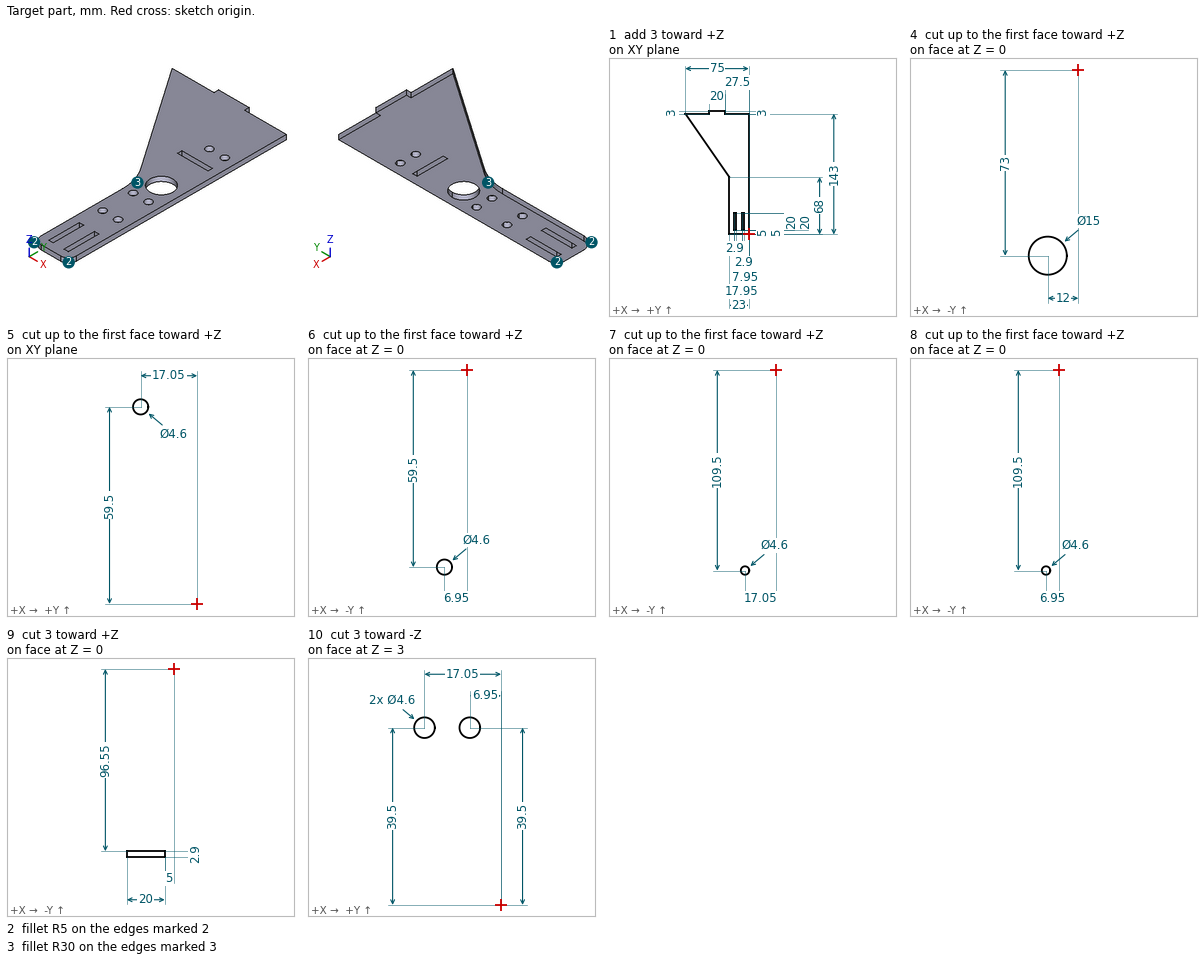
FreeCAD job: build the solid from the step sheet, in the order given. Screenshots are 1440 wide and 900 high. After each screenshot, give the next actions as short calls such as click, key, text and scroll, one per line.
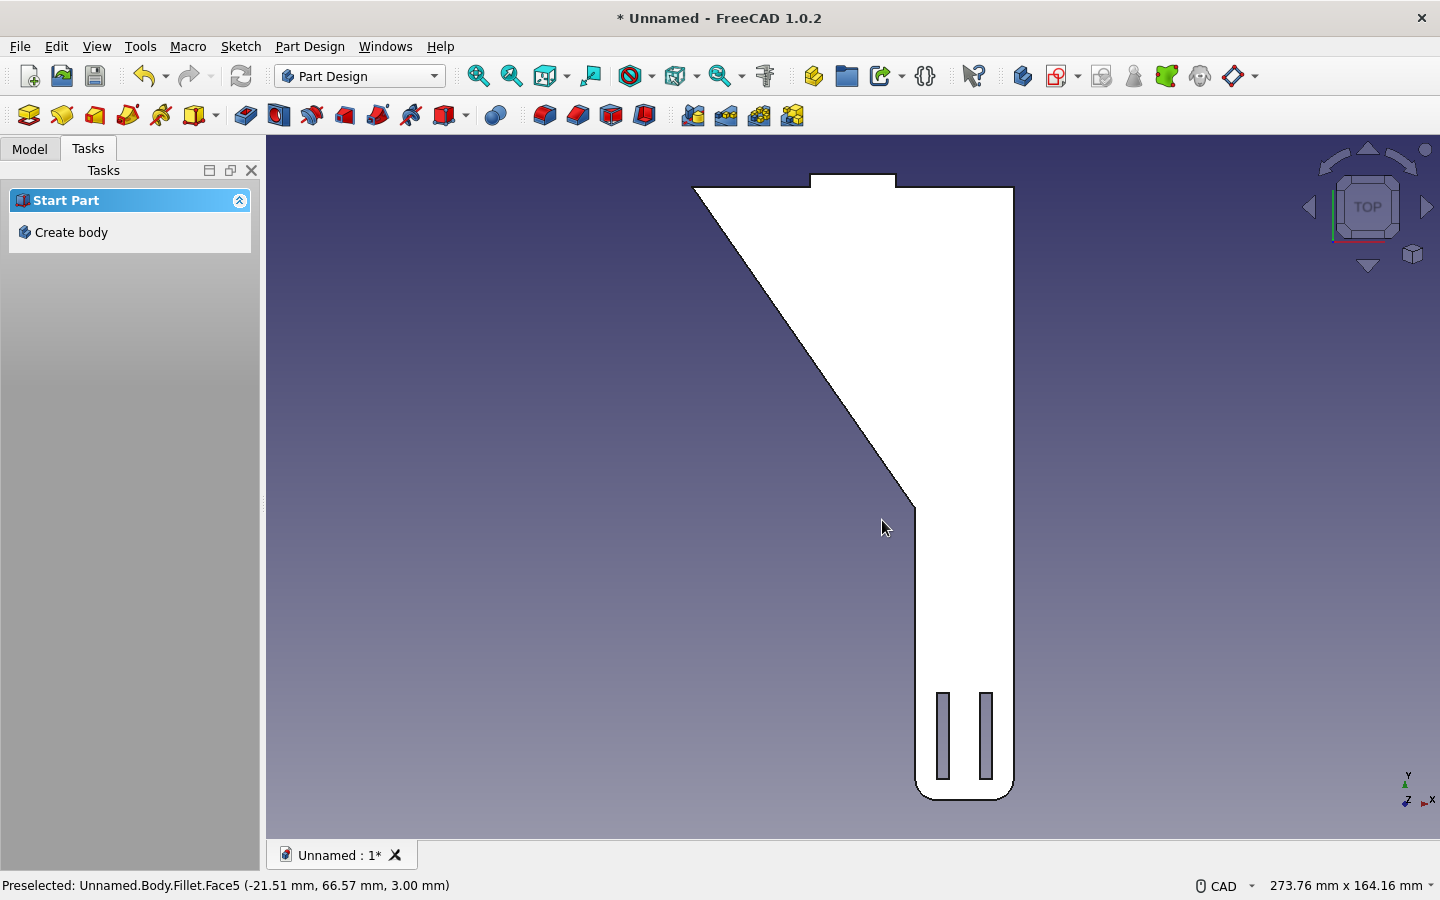
scroll(915, 507, up, 6)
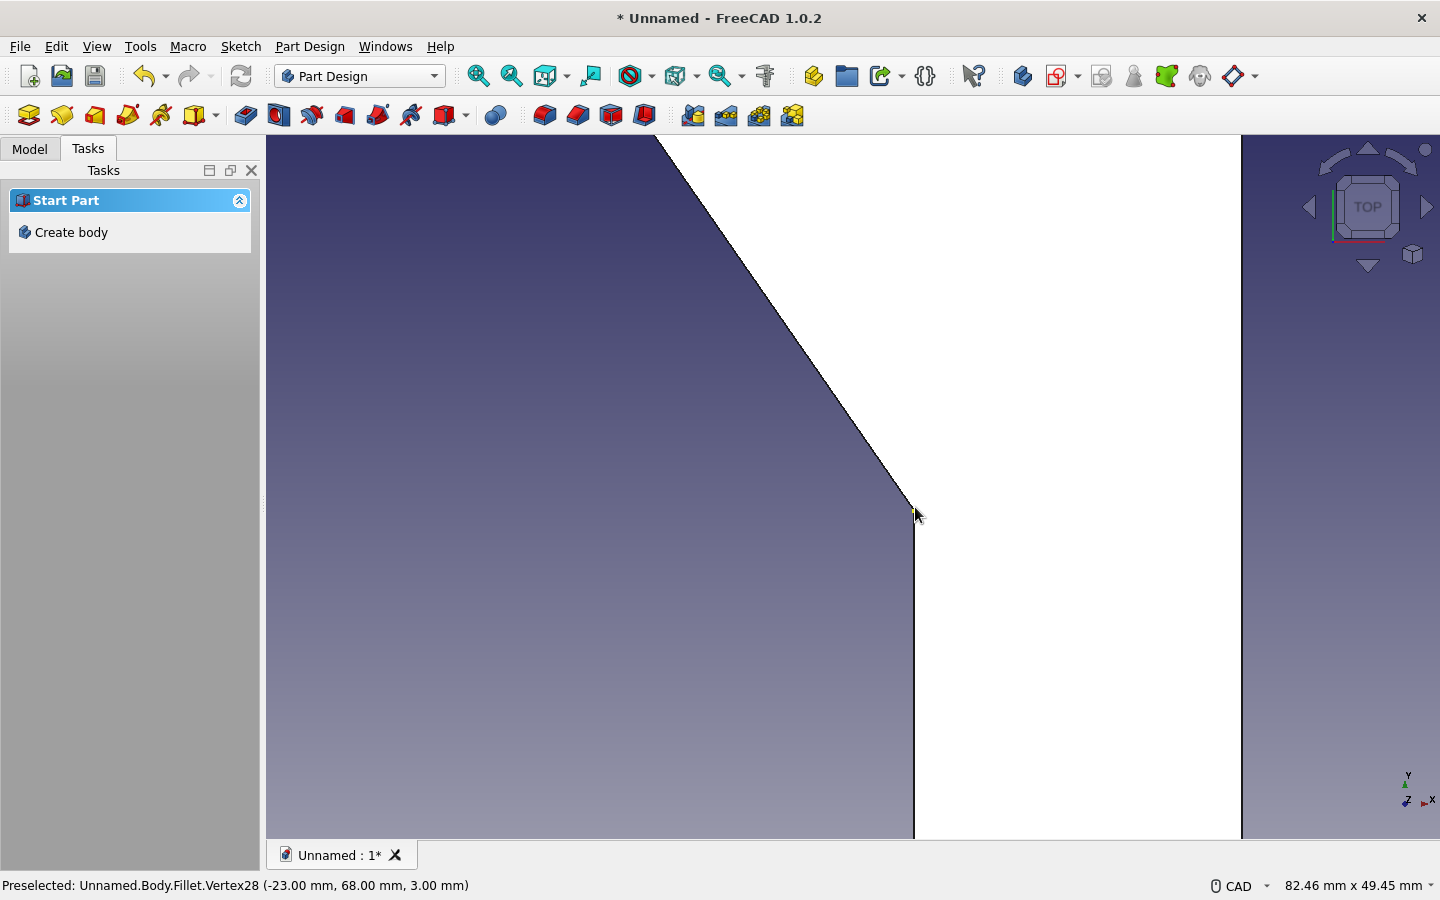
click(479, 76)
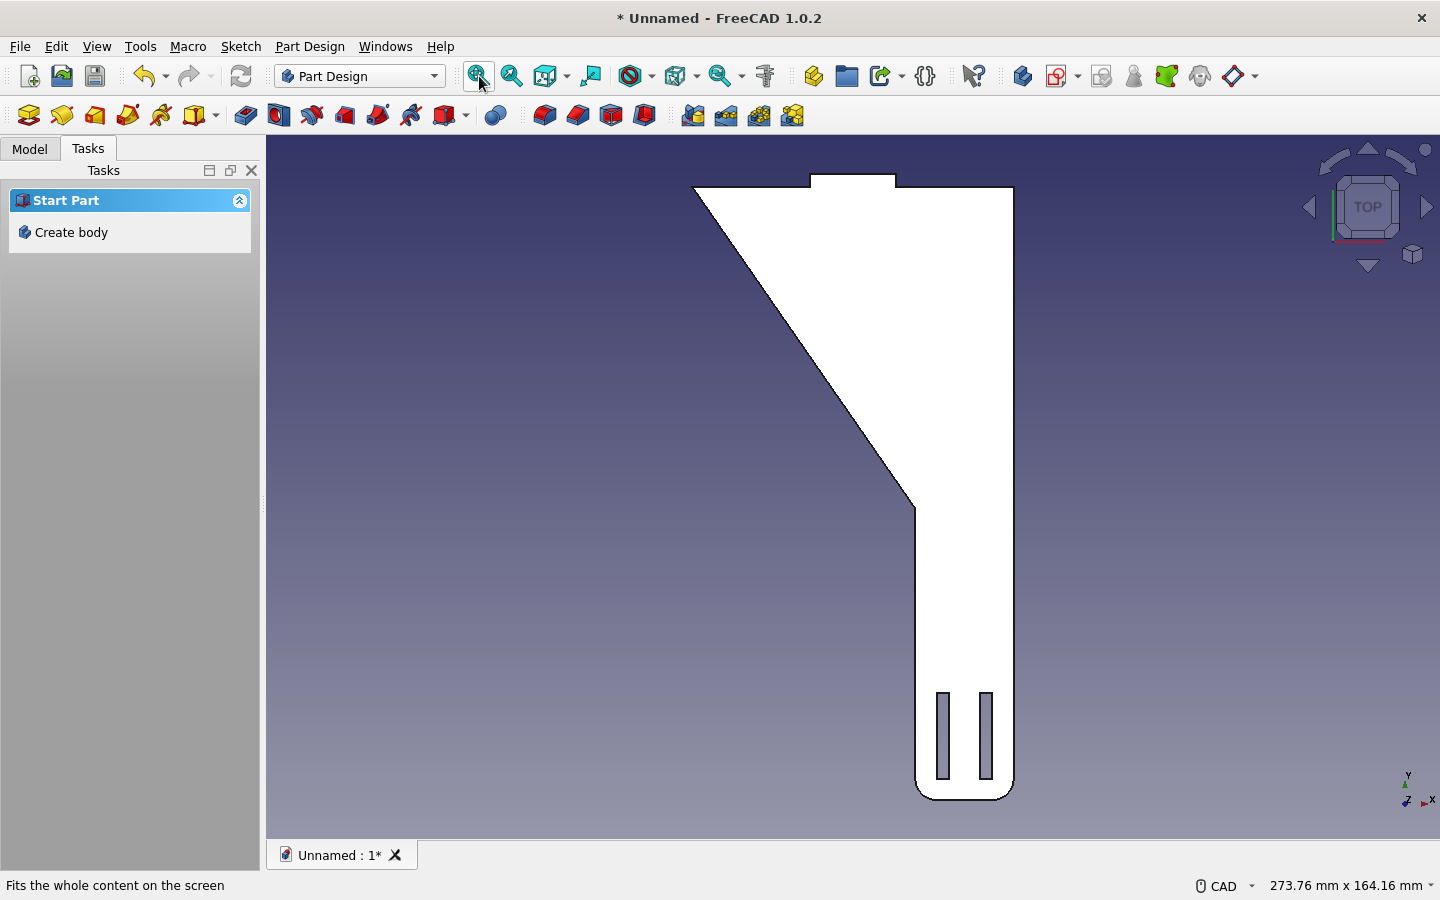
key(1)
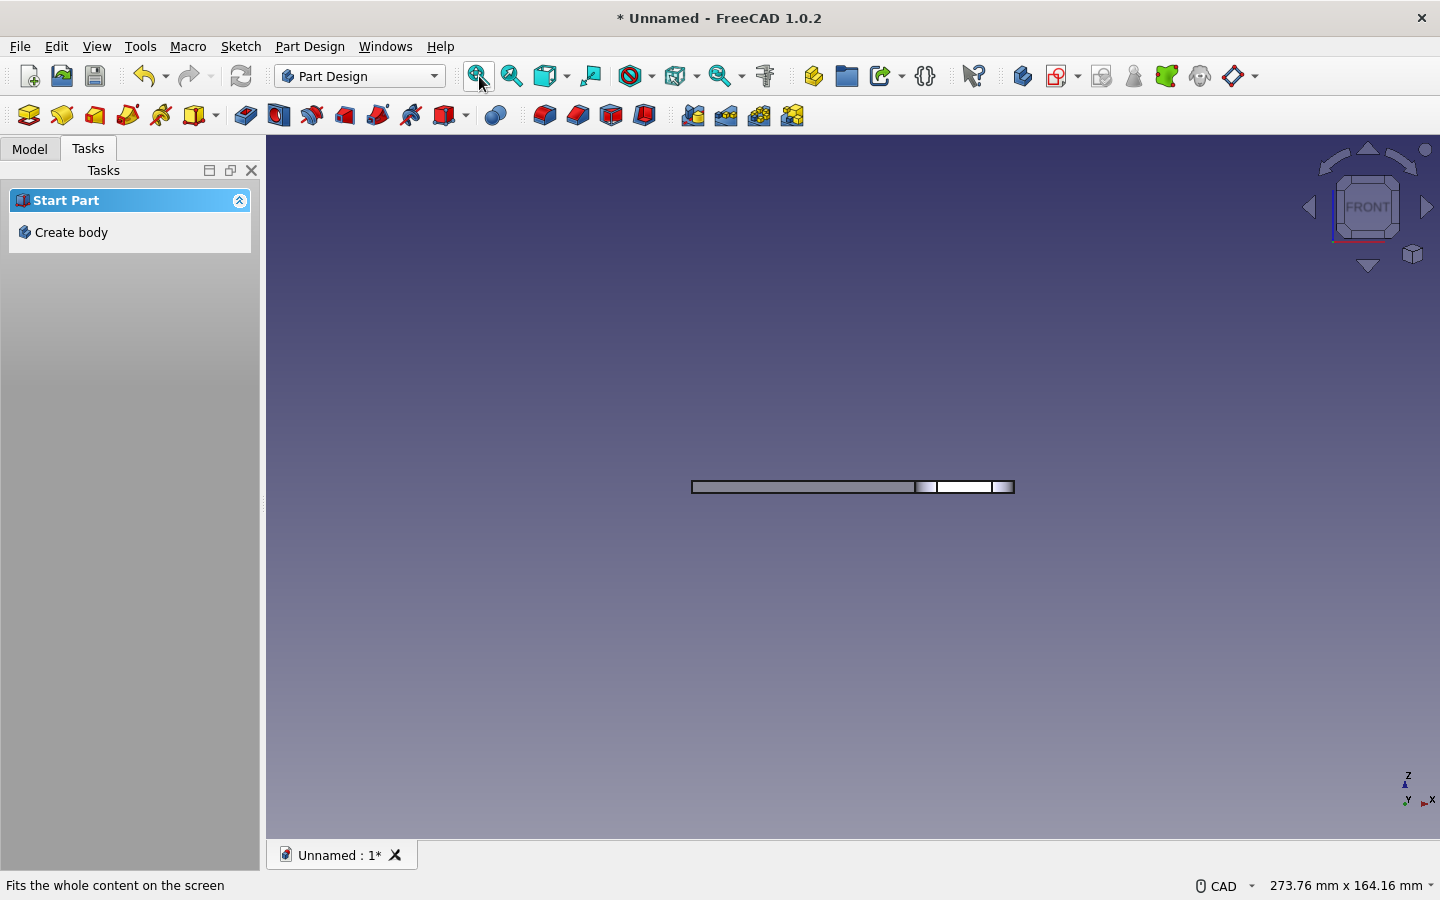
key(v)
key(f)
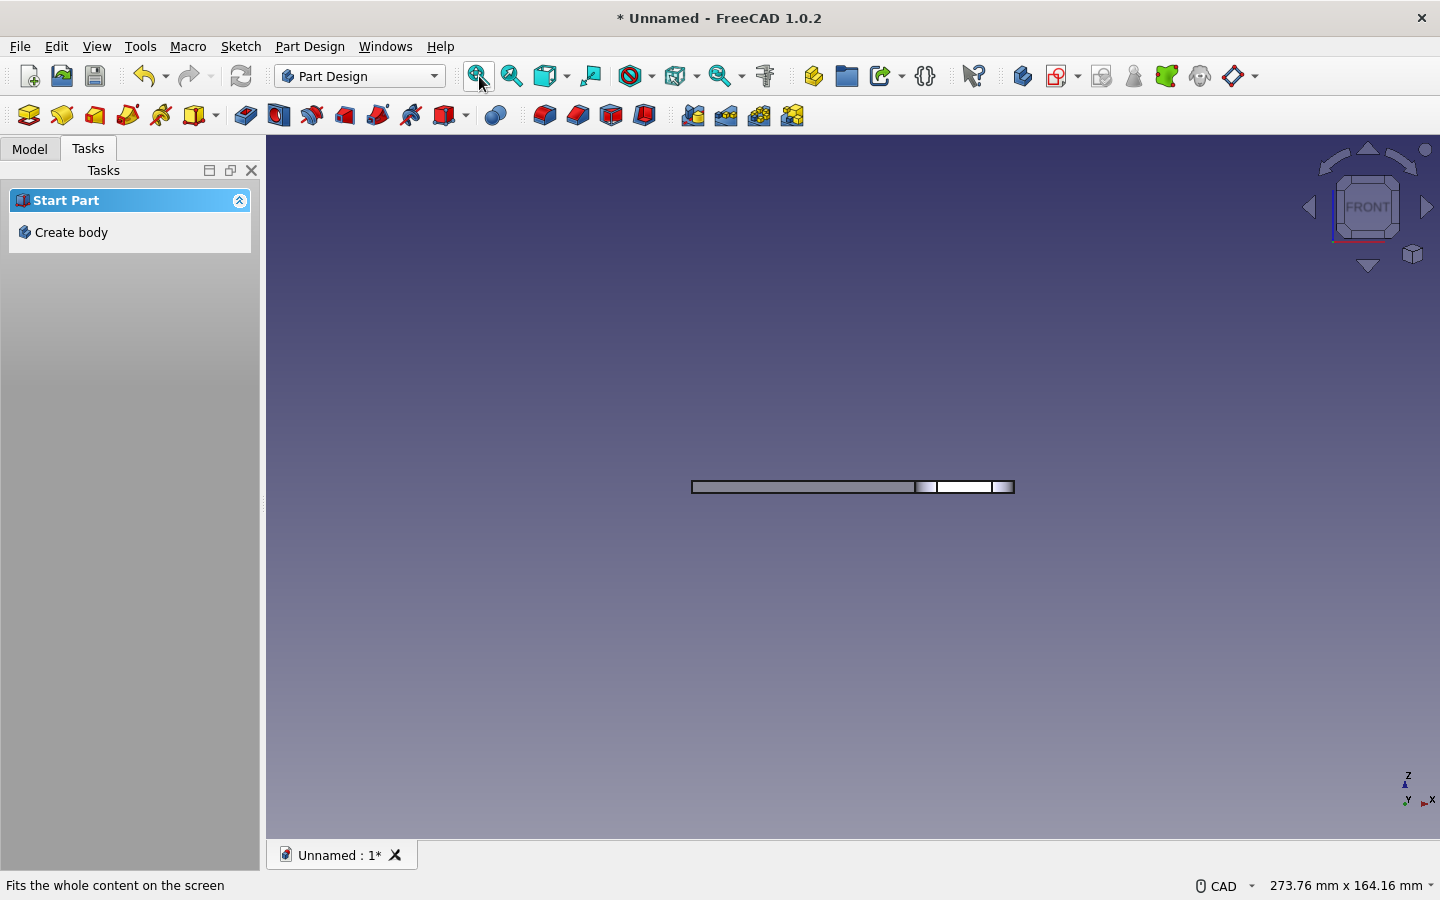
scroll(915, 486, up, 6)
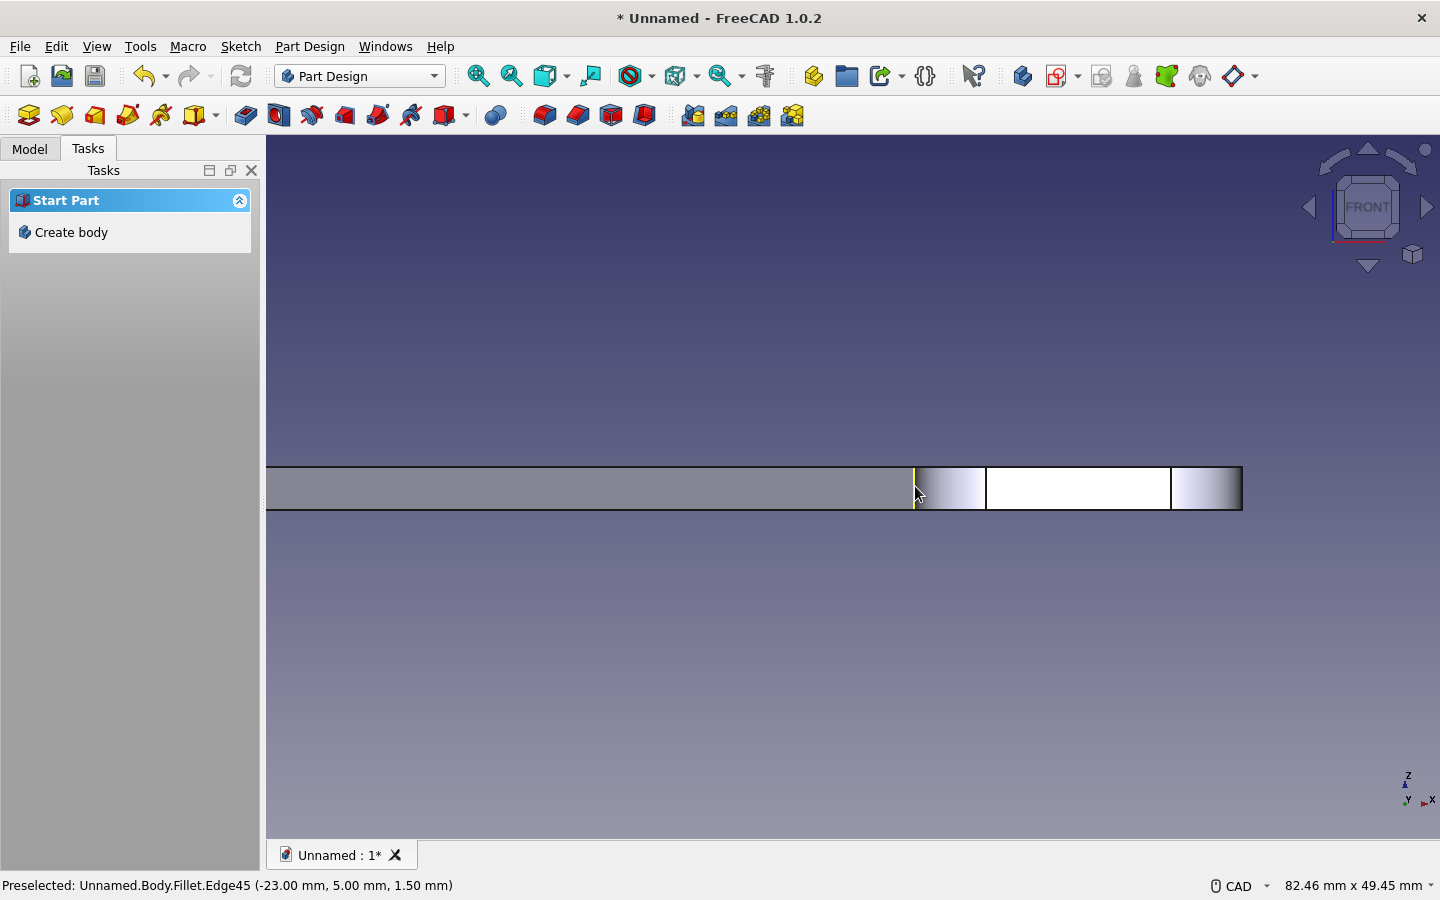
key(v)
key(f)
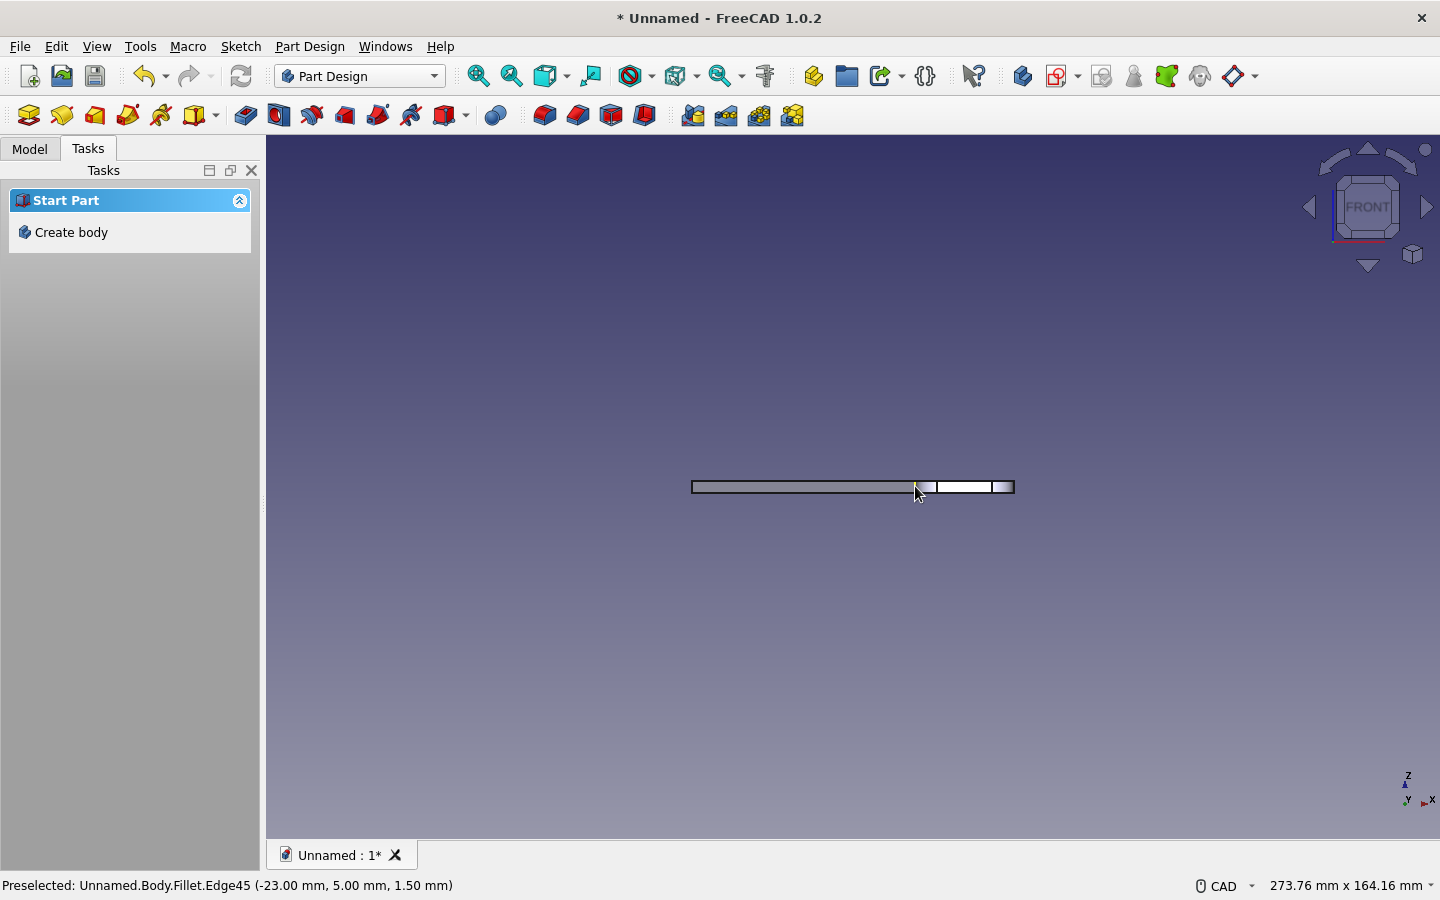
key(3)